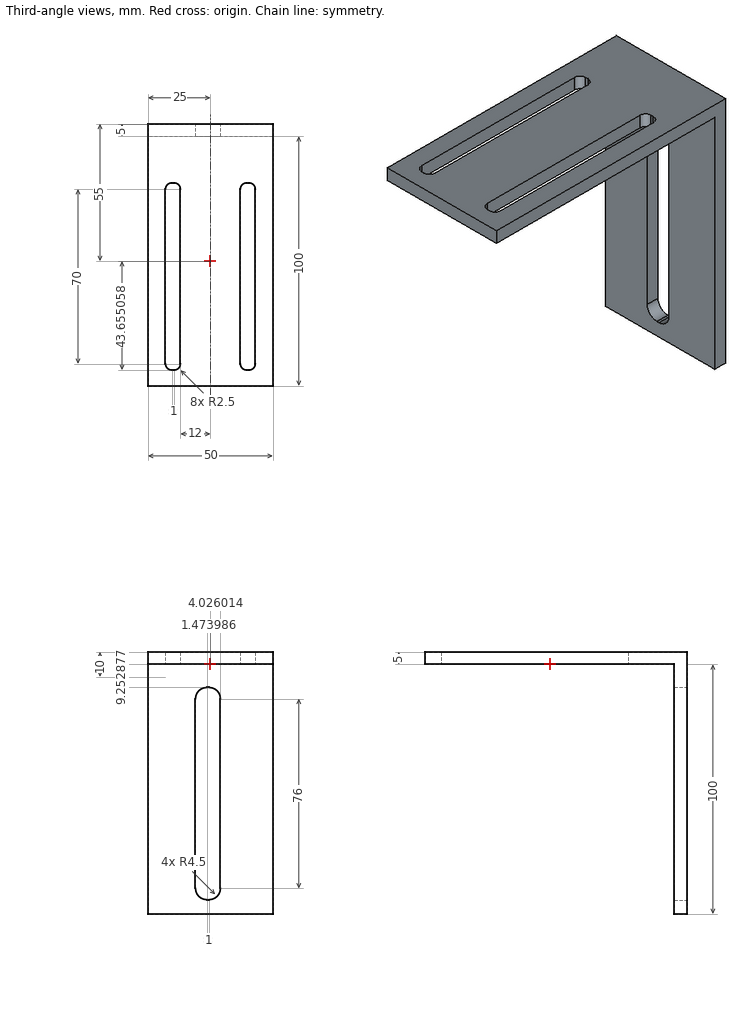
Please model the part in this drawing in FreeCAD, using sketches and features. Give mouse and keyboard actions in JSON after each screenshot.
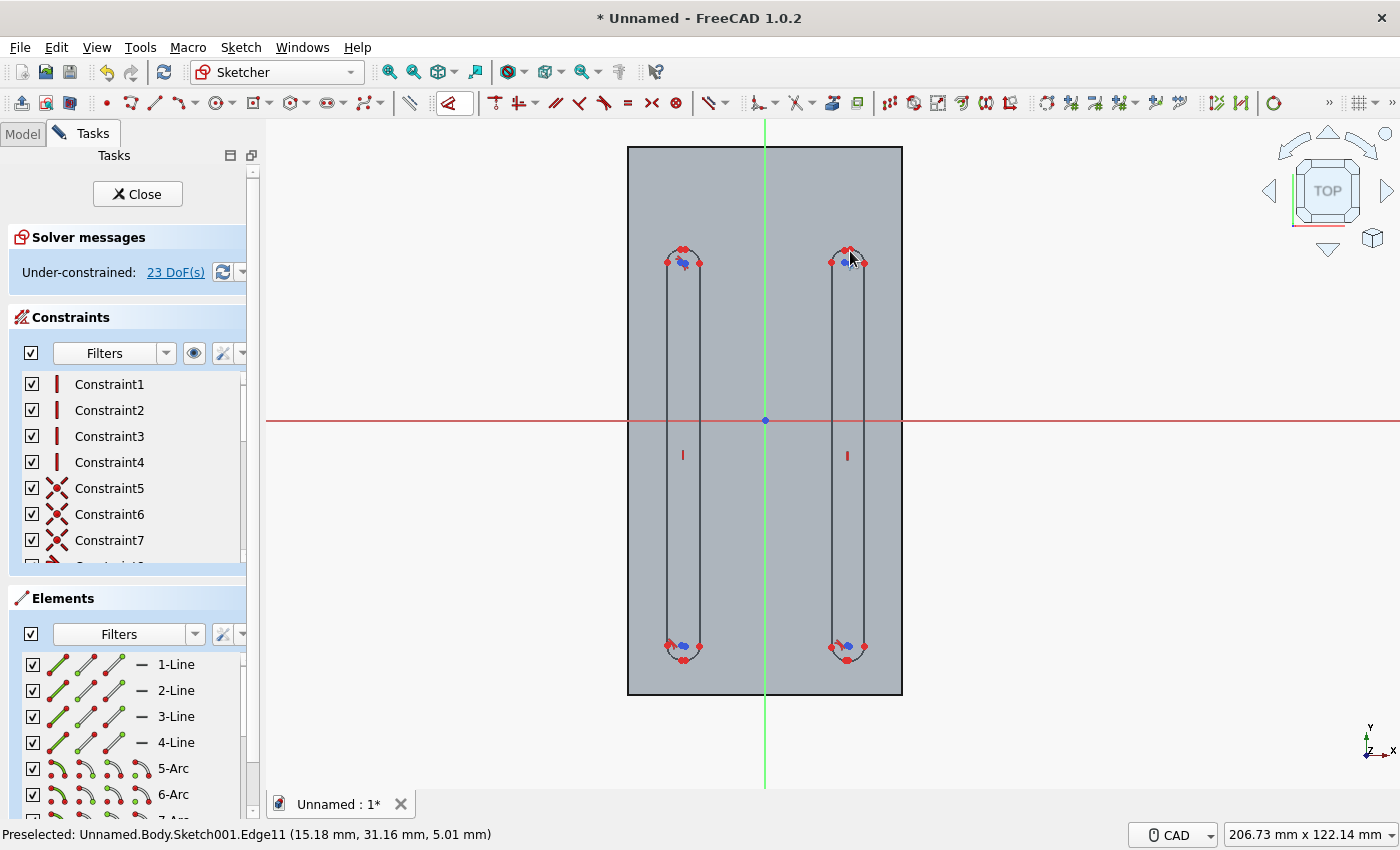
{"action": "scroll", "coordinate": [839, 251], "scroll_direction": "up", "scroll_amount": 5}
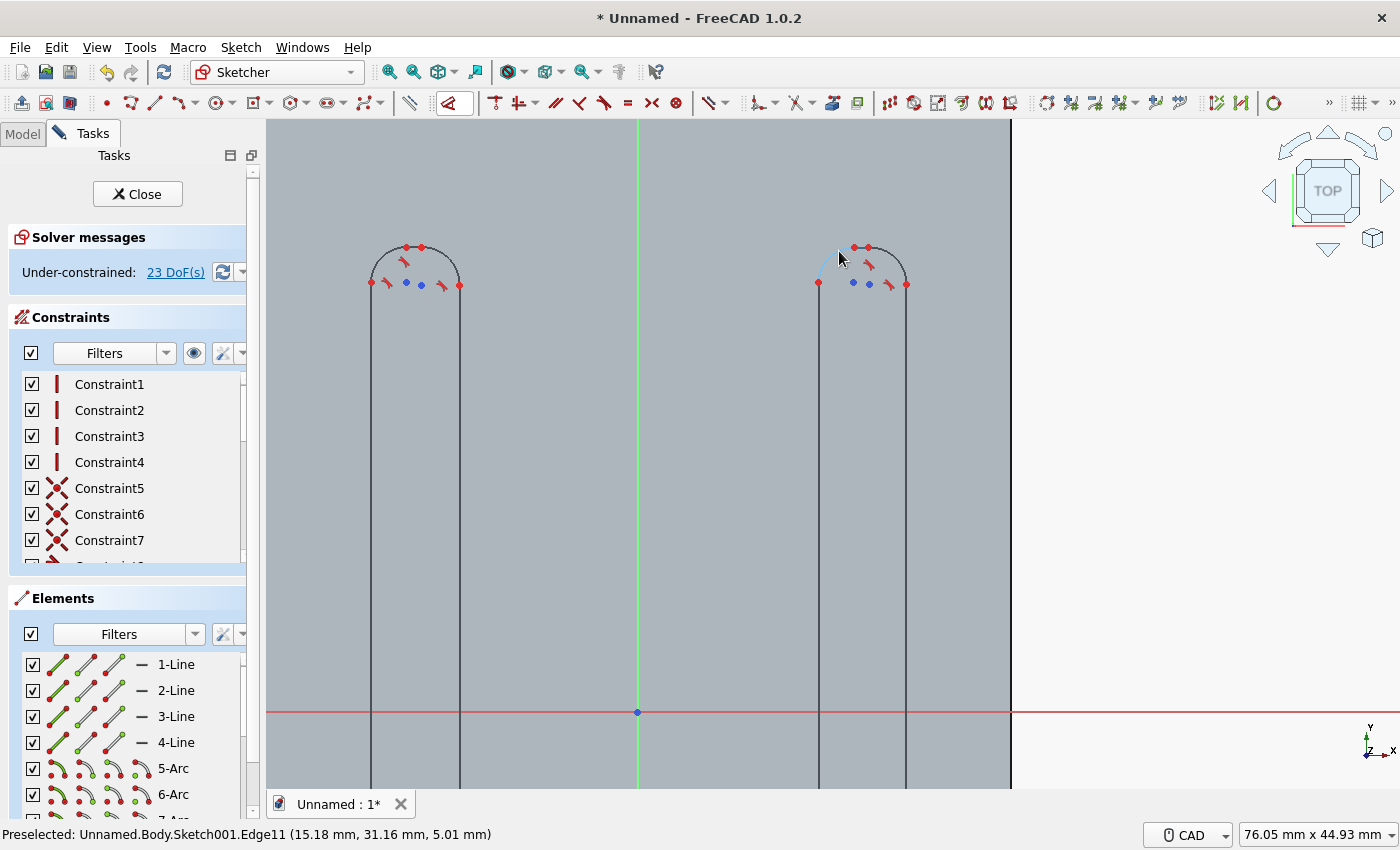
{"action": "left_click", "coordinate": [838, 252]}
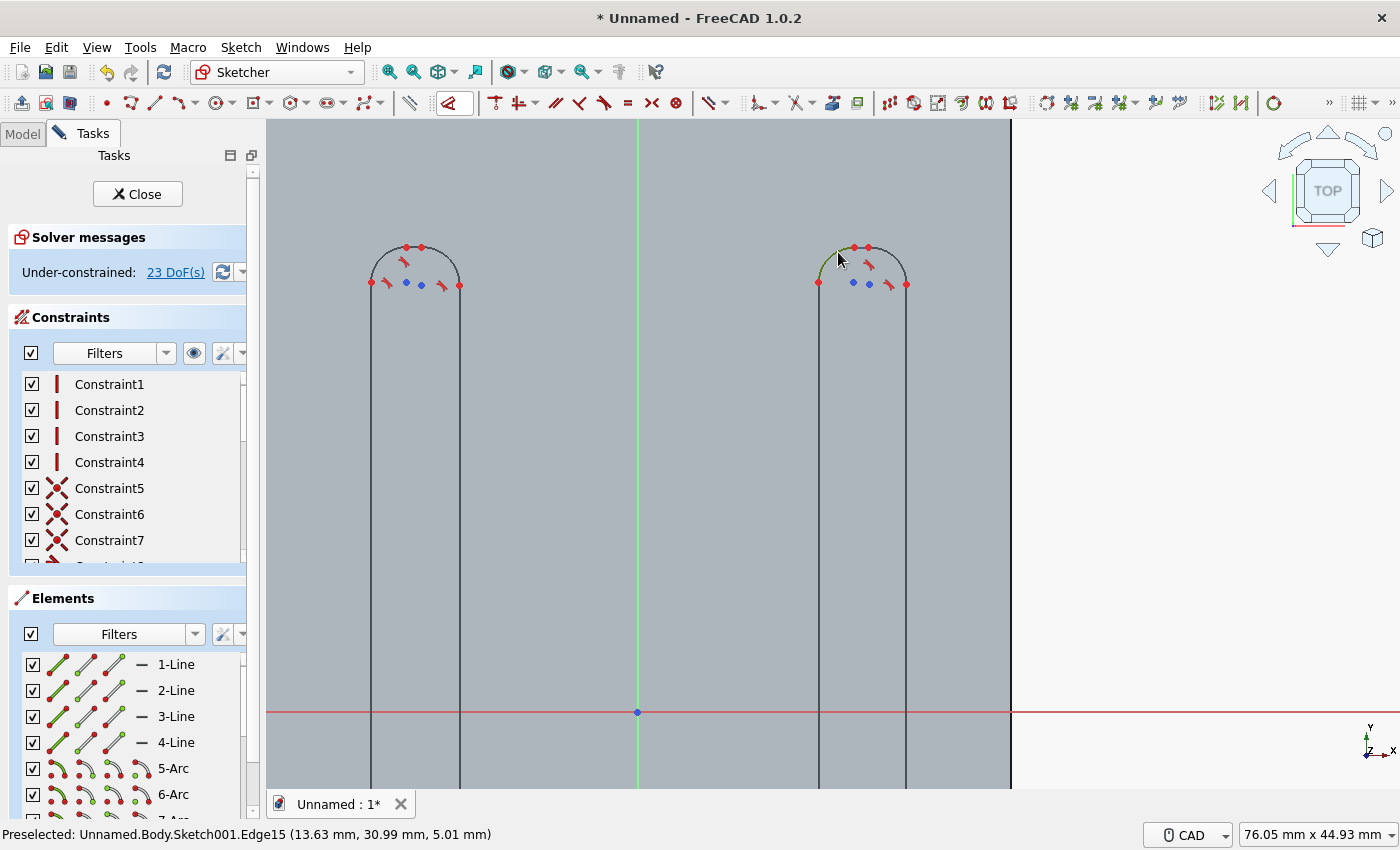
{"action": "left_click", "coordinate": [604, 104]}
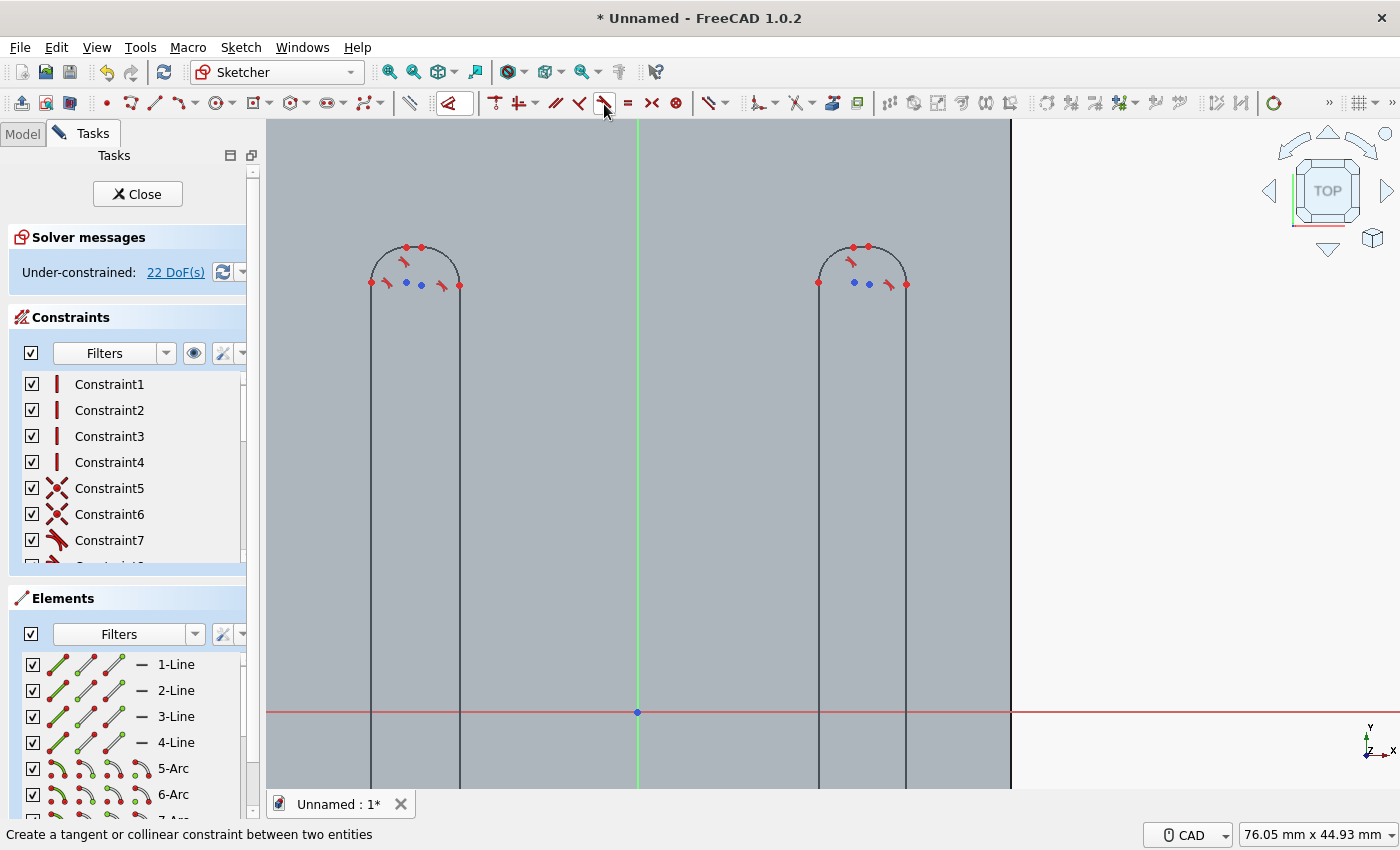
{"action": "left_click", "coordinate": [819, 596]}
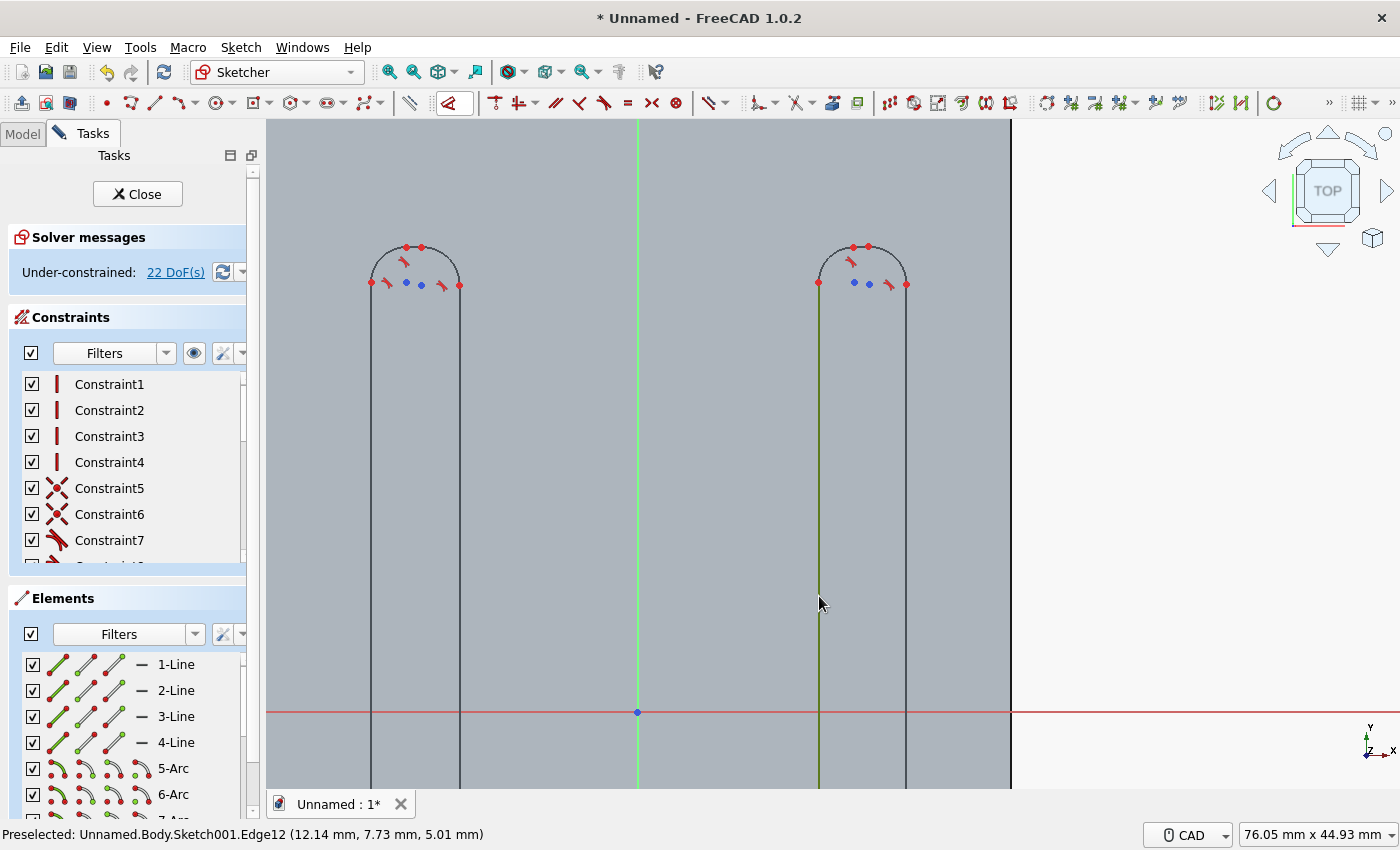
{"action": "left_click", "coordinate": [838, 251]}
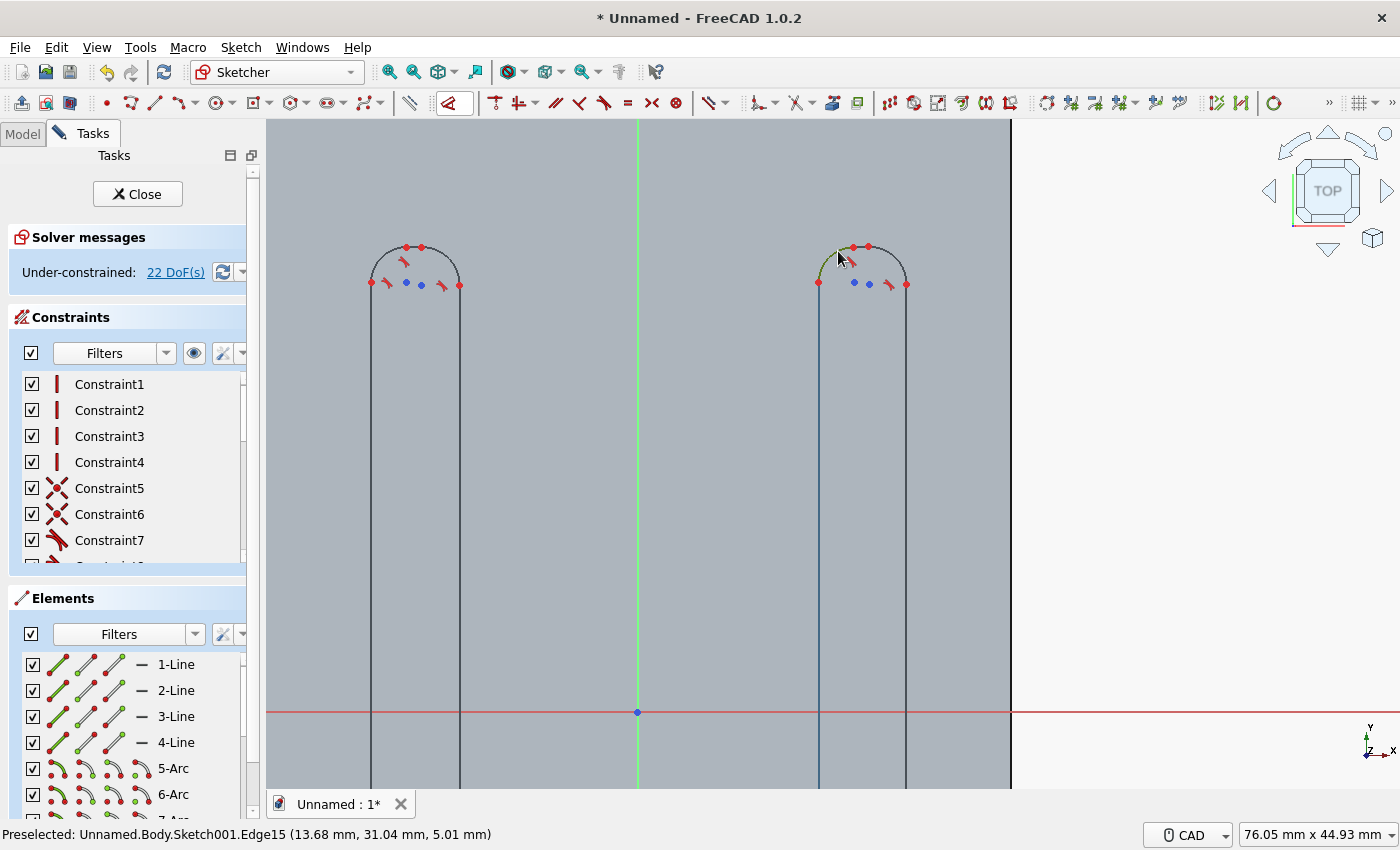
{"action": "left_click", "coordinate": [604, 104]}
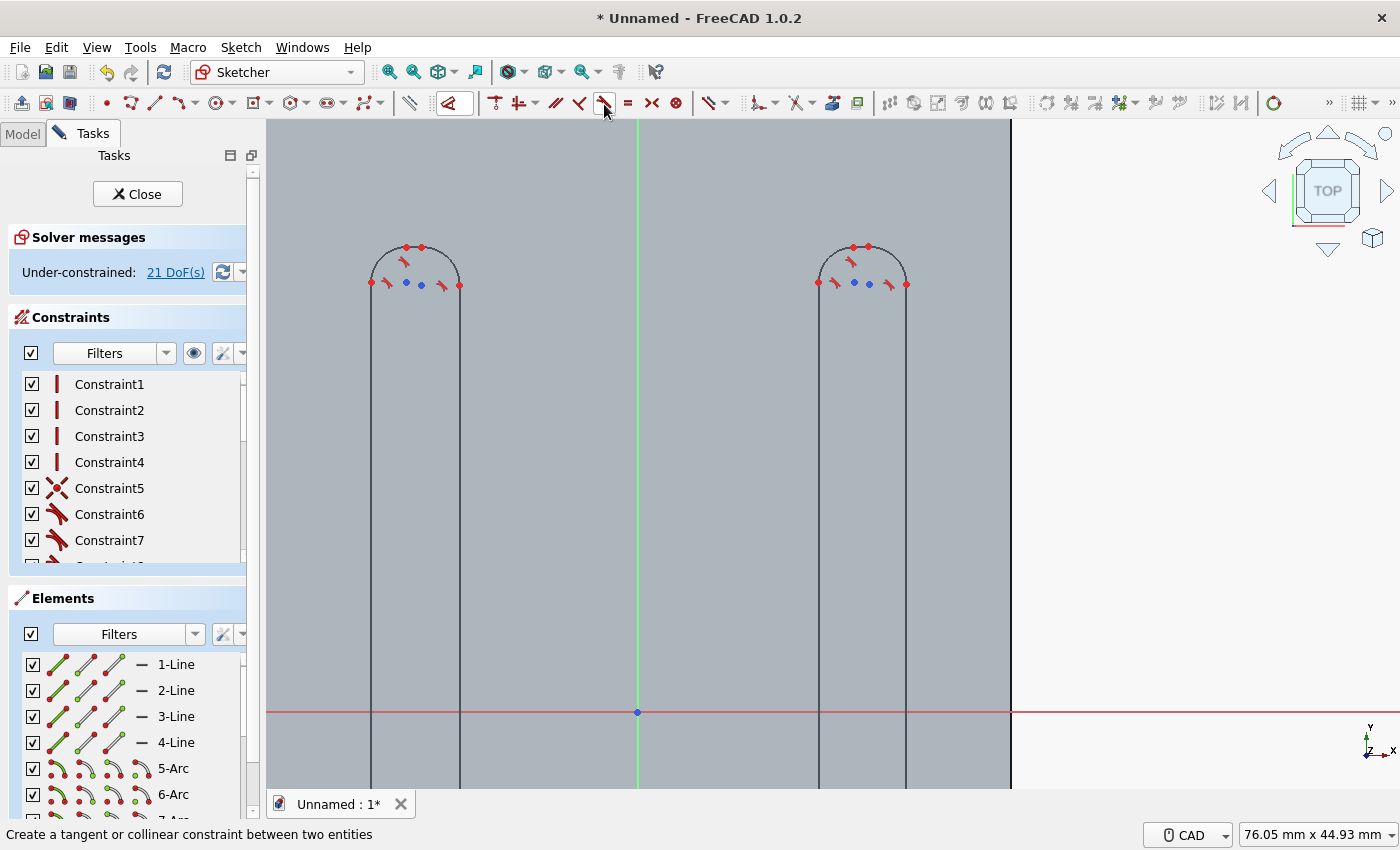
{"action": "left_click", "coordinate": [819, 596]}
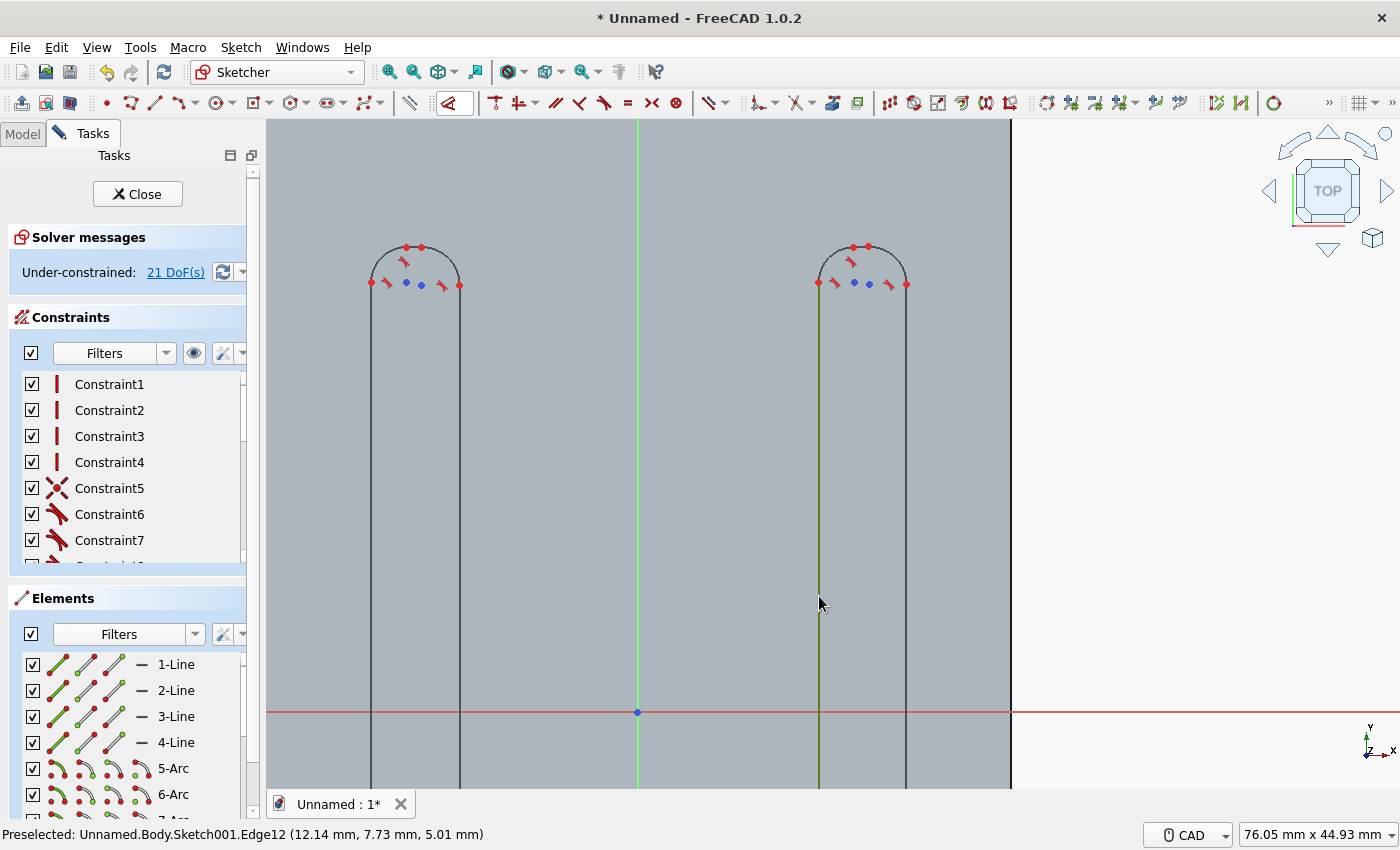
{"action": "scroll", "coordinate": [838, 250], "scroll_direction": "down", "scroll_amount": 5}